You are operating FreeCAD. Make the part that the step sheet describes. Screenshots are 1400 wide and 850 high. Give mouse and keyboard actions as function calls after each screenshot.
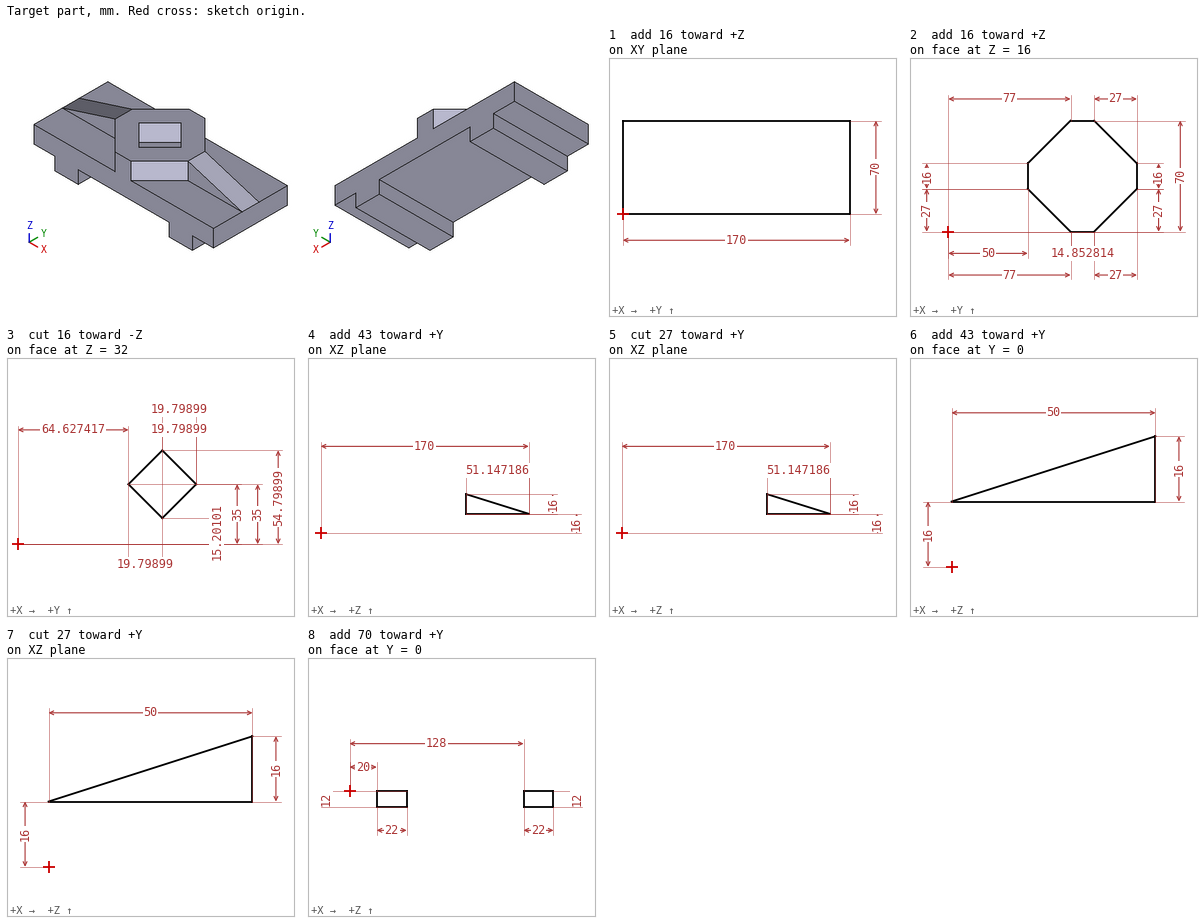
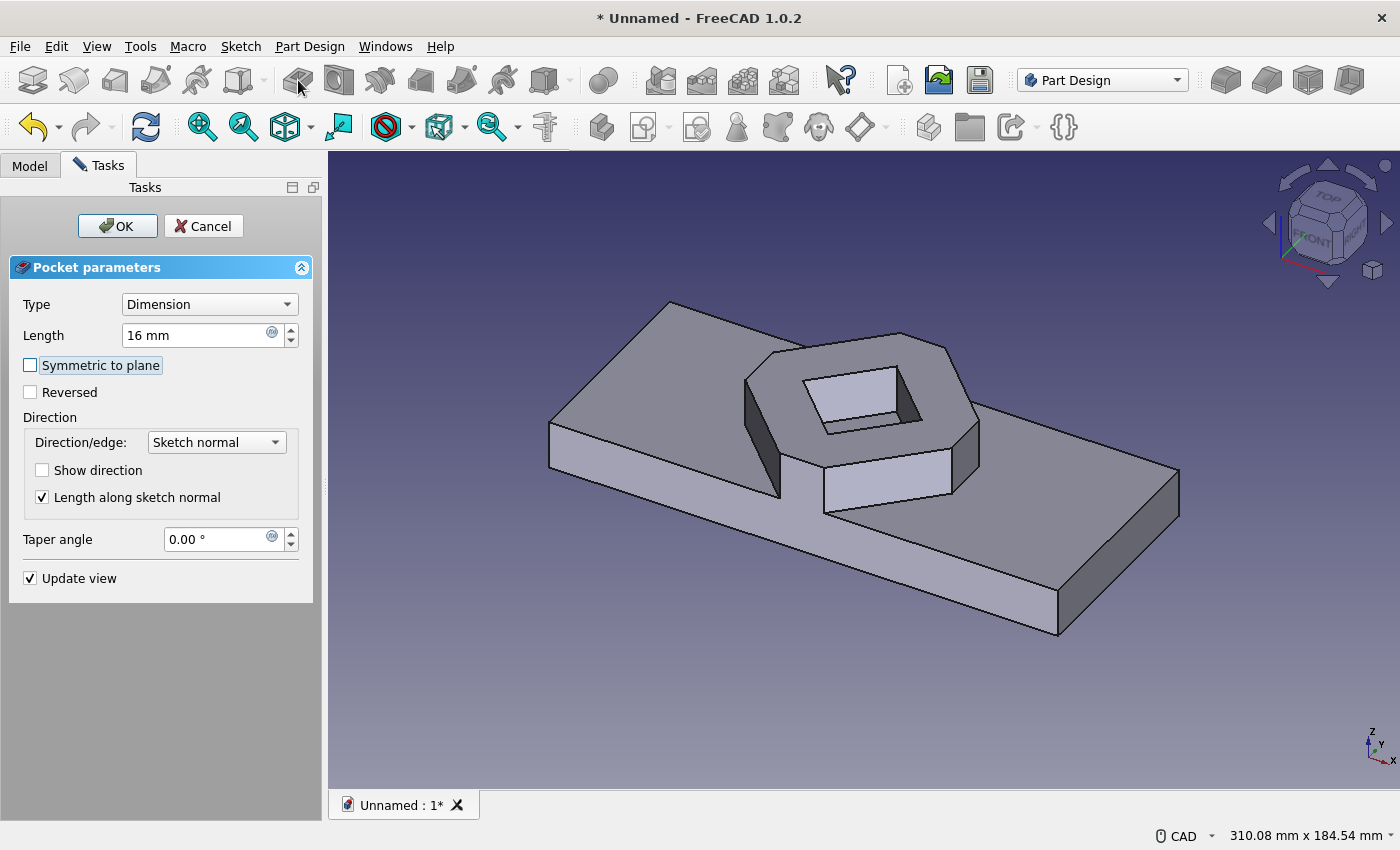
click(118, 226)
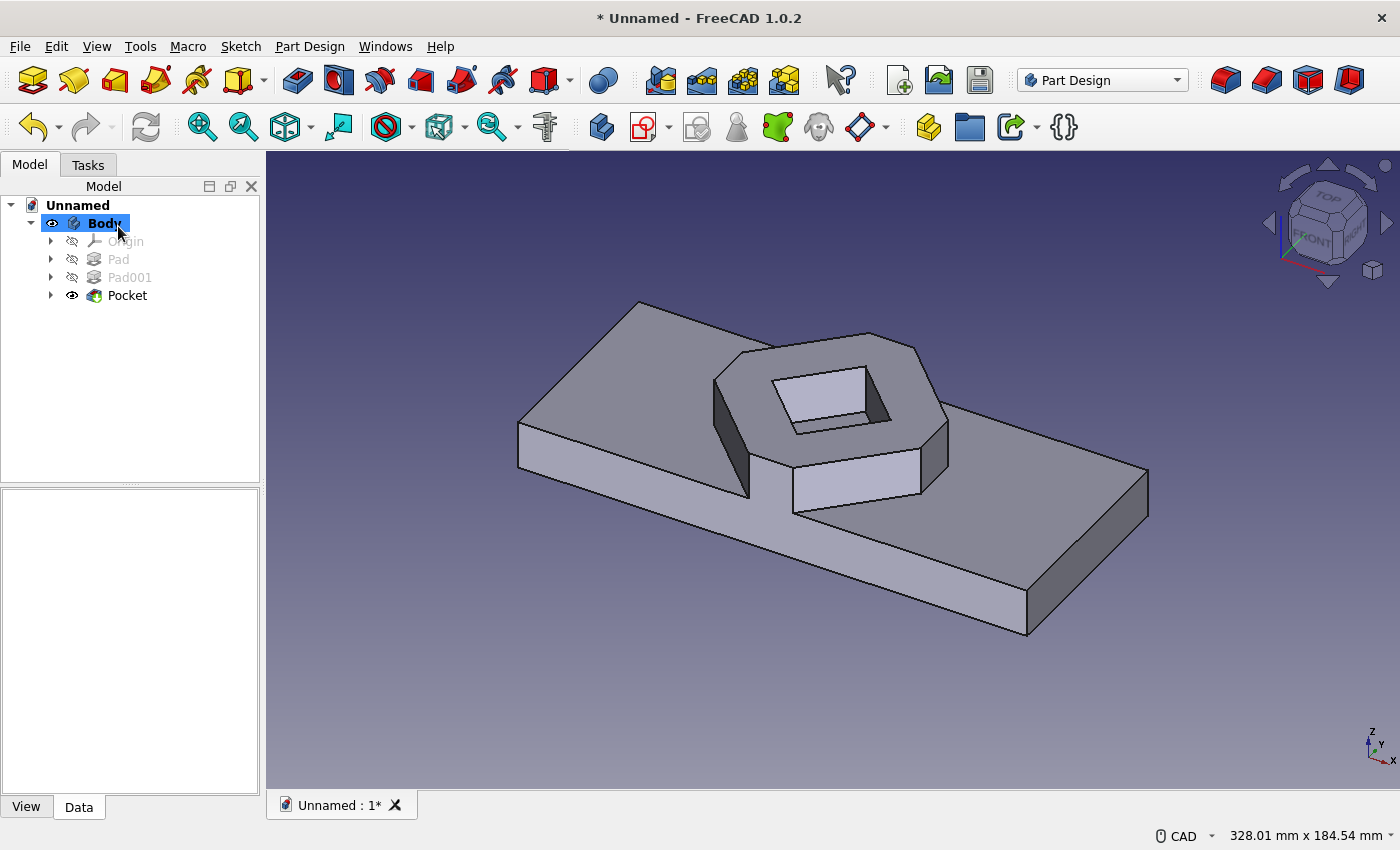
click(642, 128)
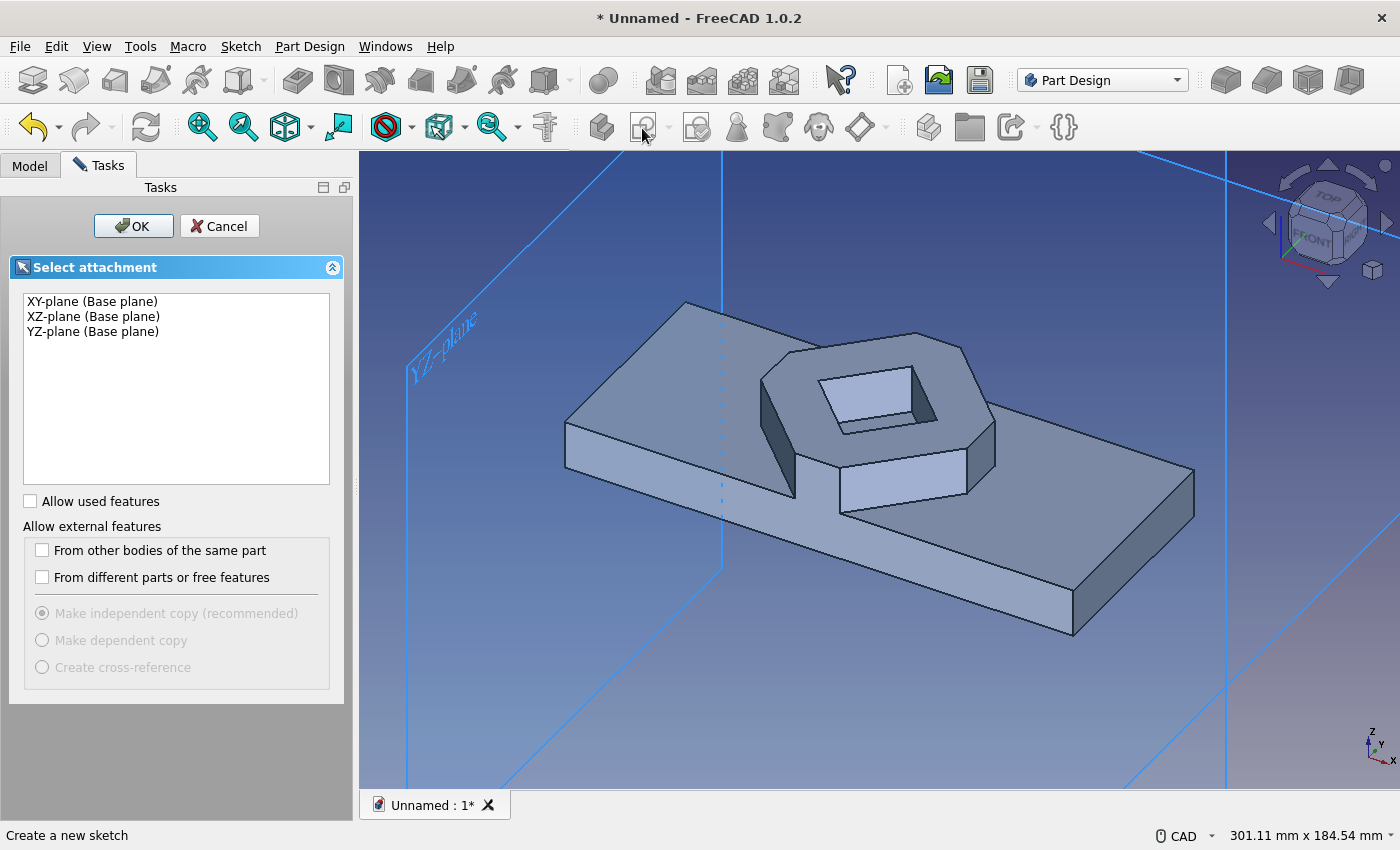
click(84, 316)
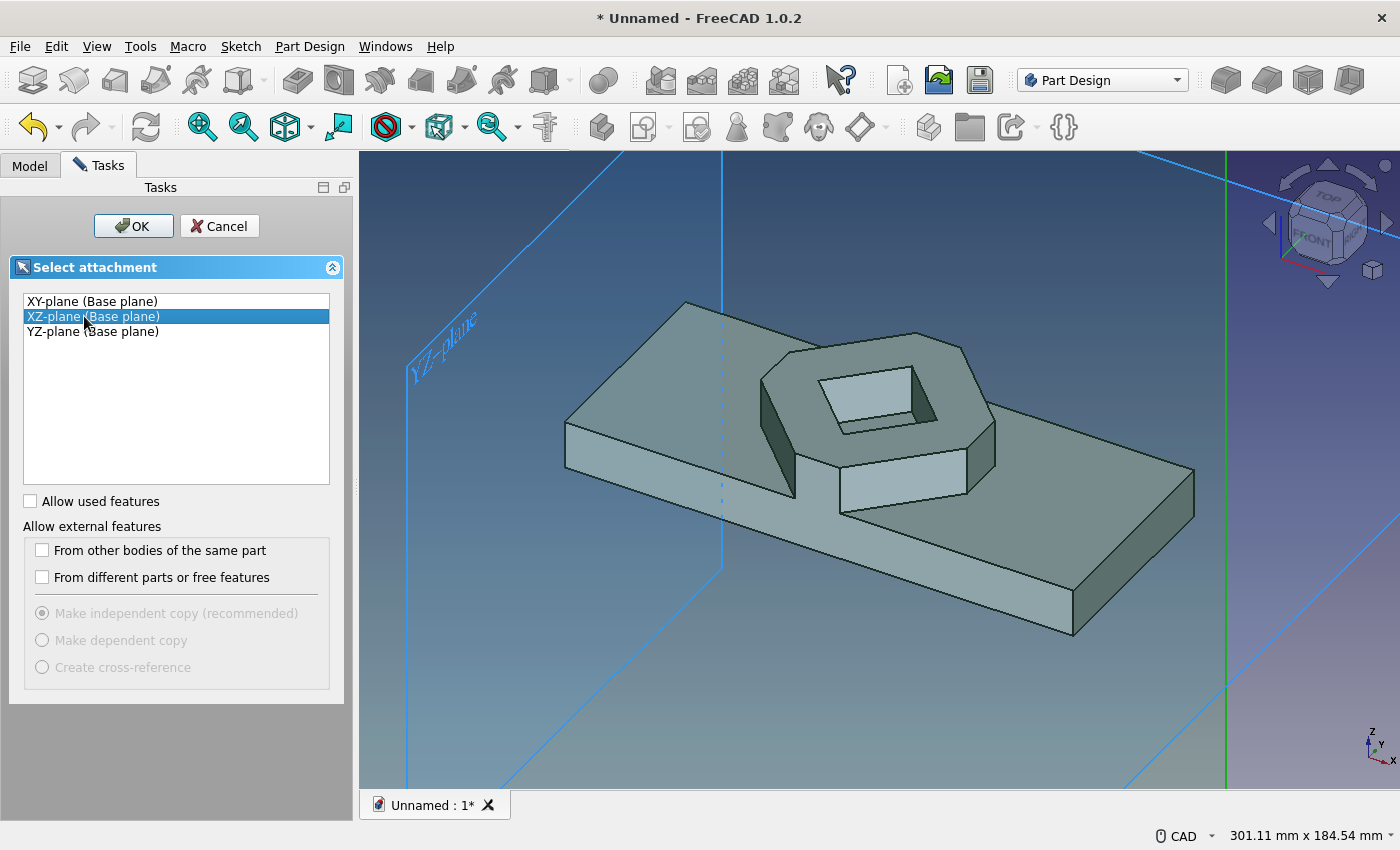
click(134, 226)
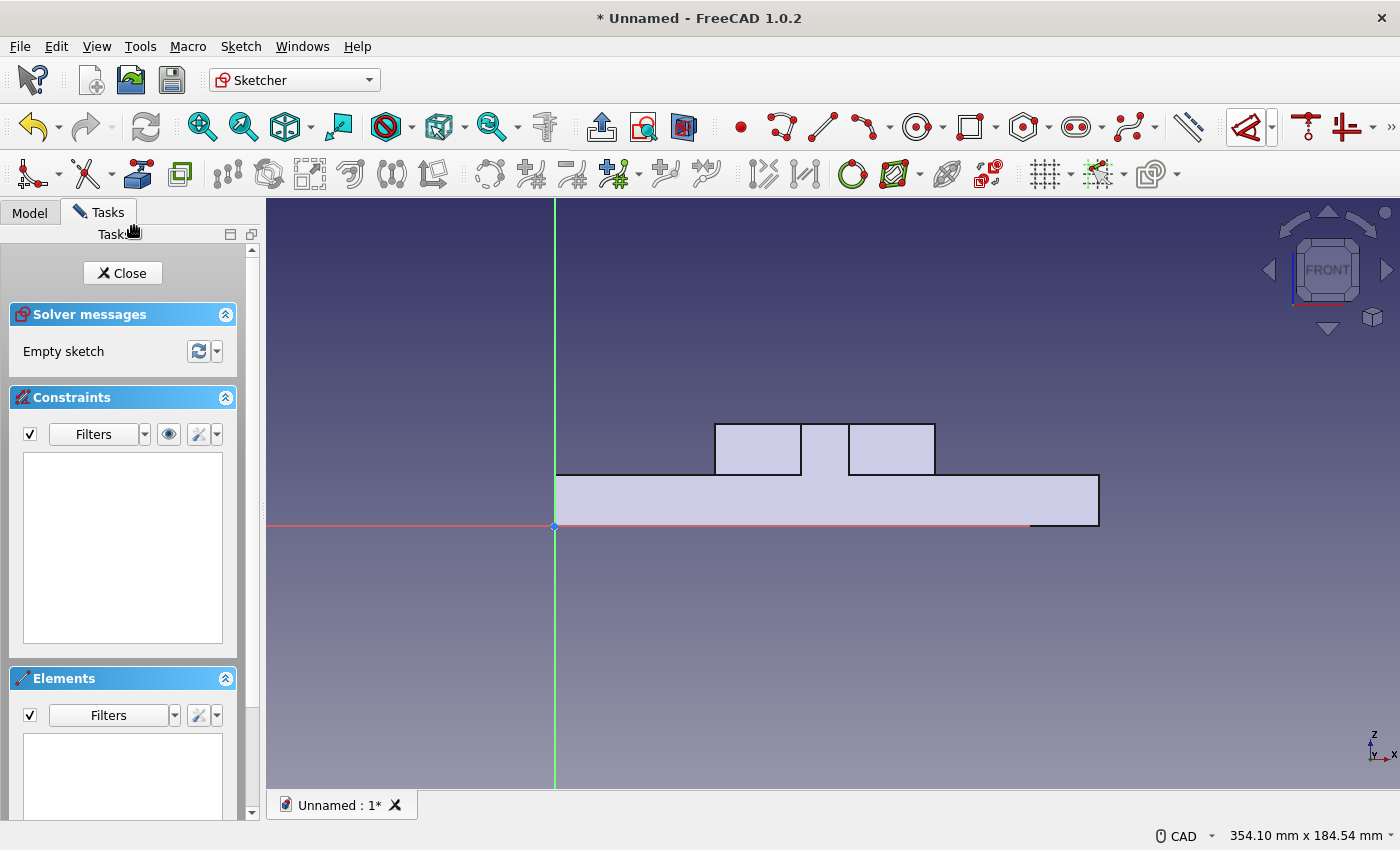
scroll(1100, 435, up, 7)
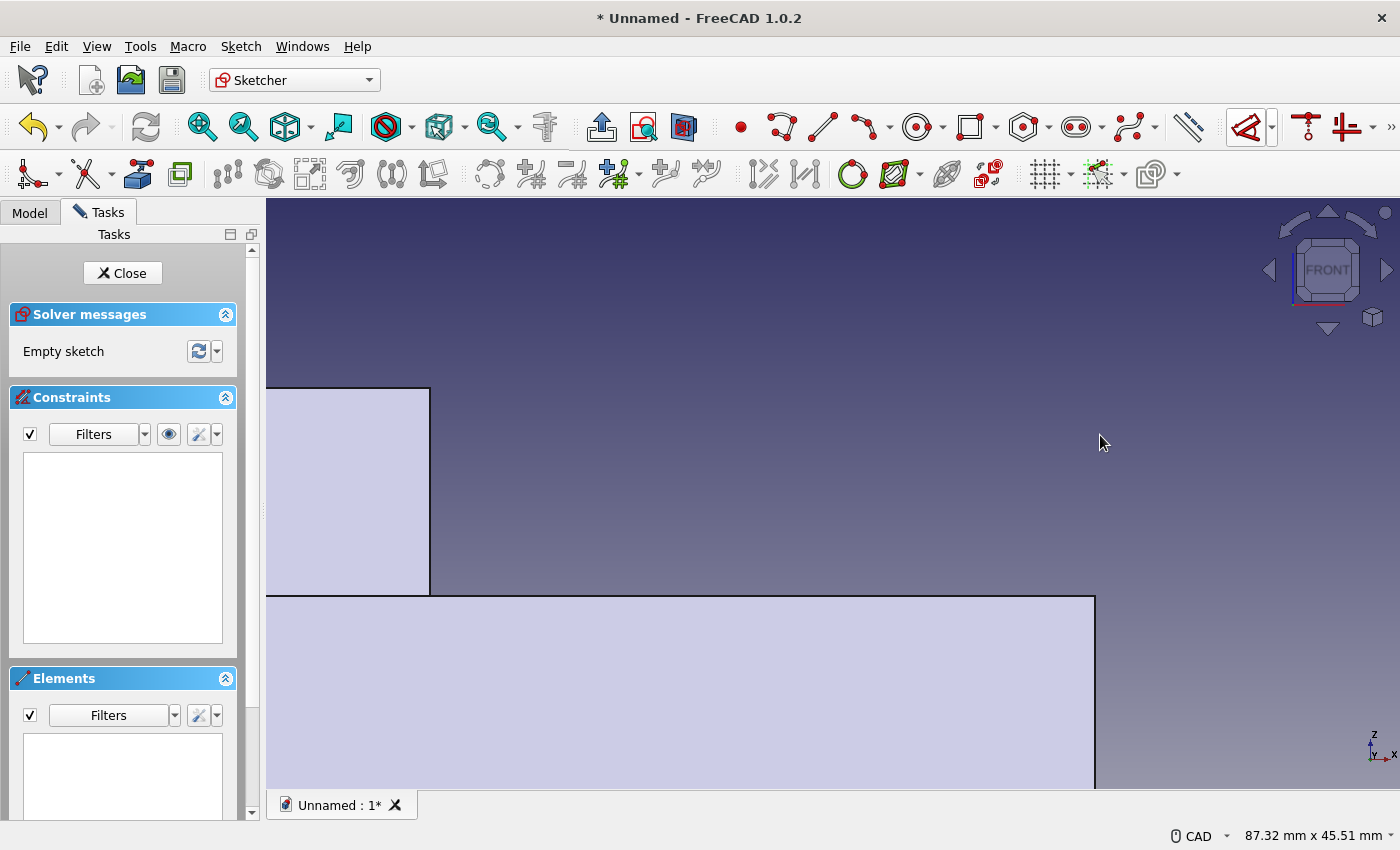
key(g)
key(m)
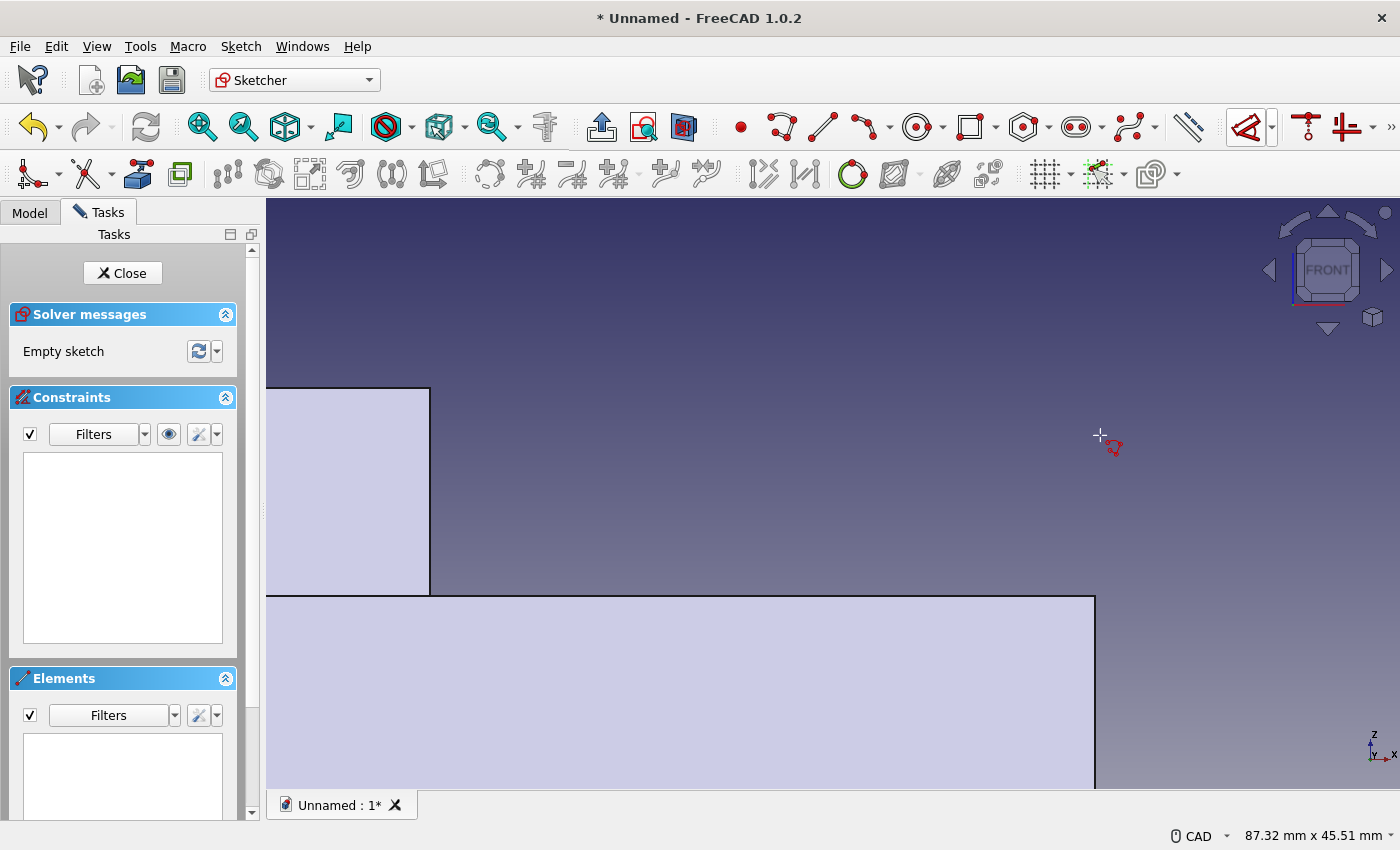
click(430, 596)
click(1095, 596)
click(430, 388)
click(430, 597)
key(Escape)
key(Escape)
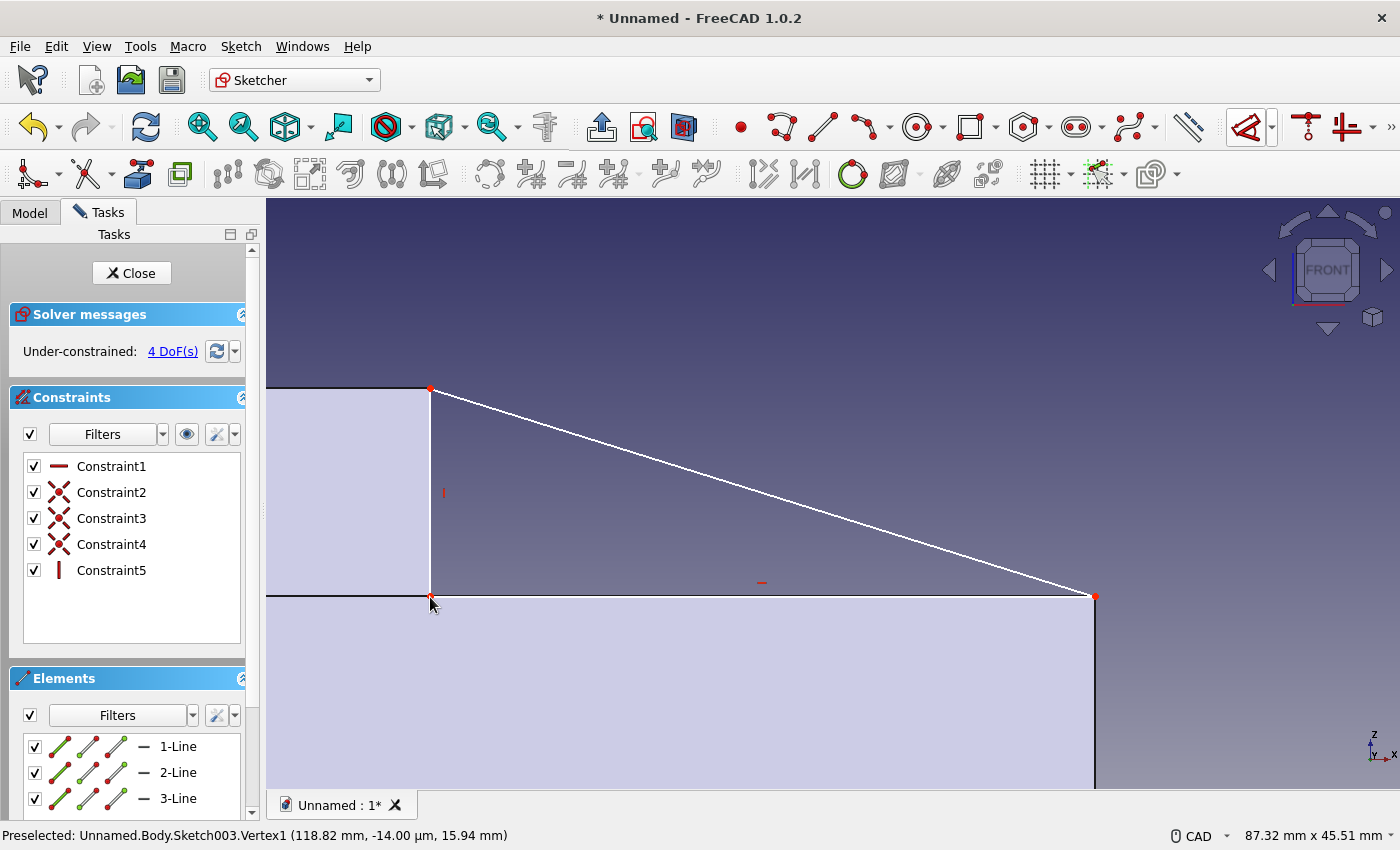
key(d)